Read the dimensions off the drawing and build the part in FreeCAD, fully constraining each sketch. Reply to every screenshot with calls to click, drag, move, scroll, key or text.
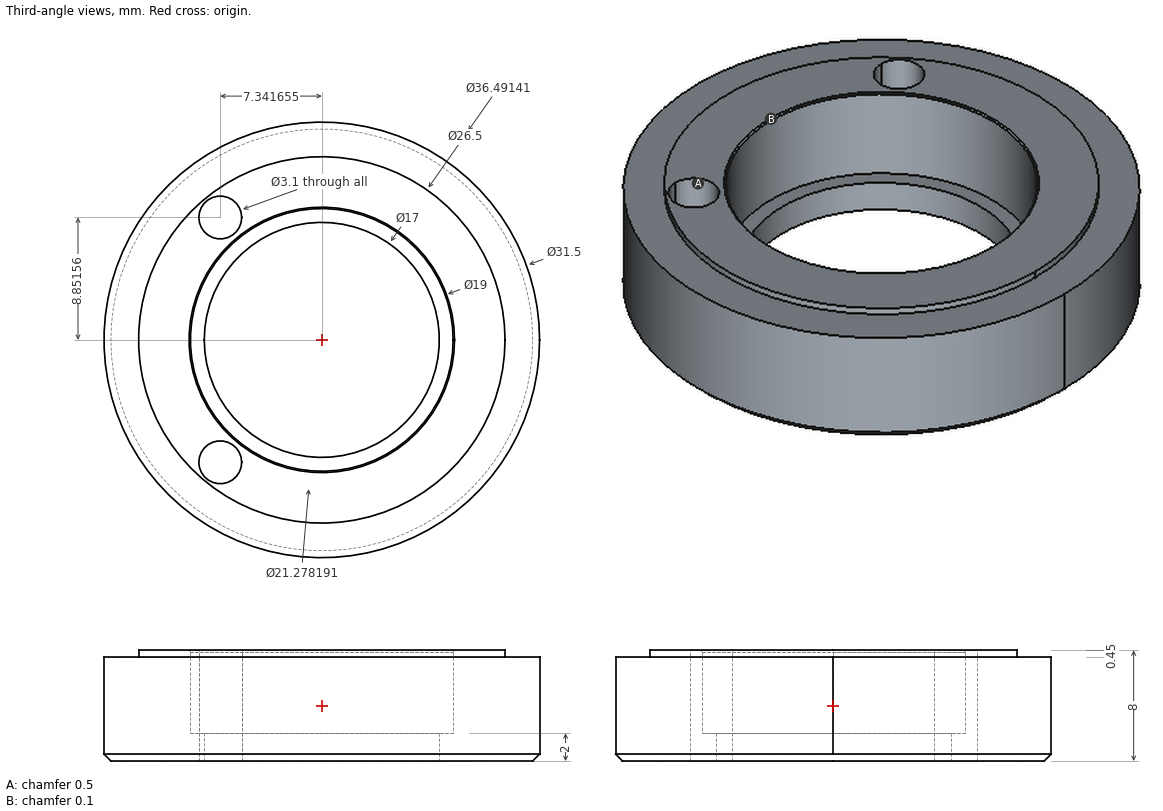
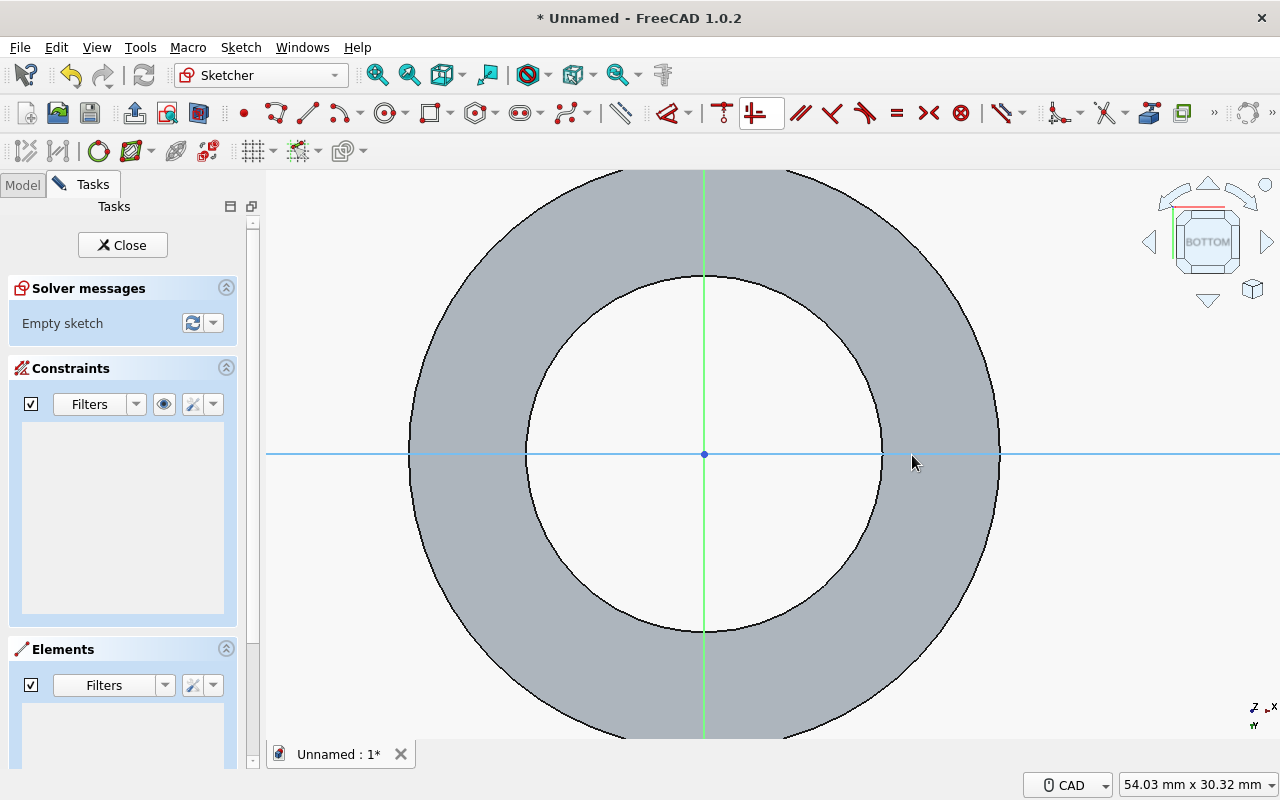
click(386, 114)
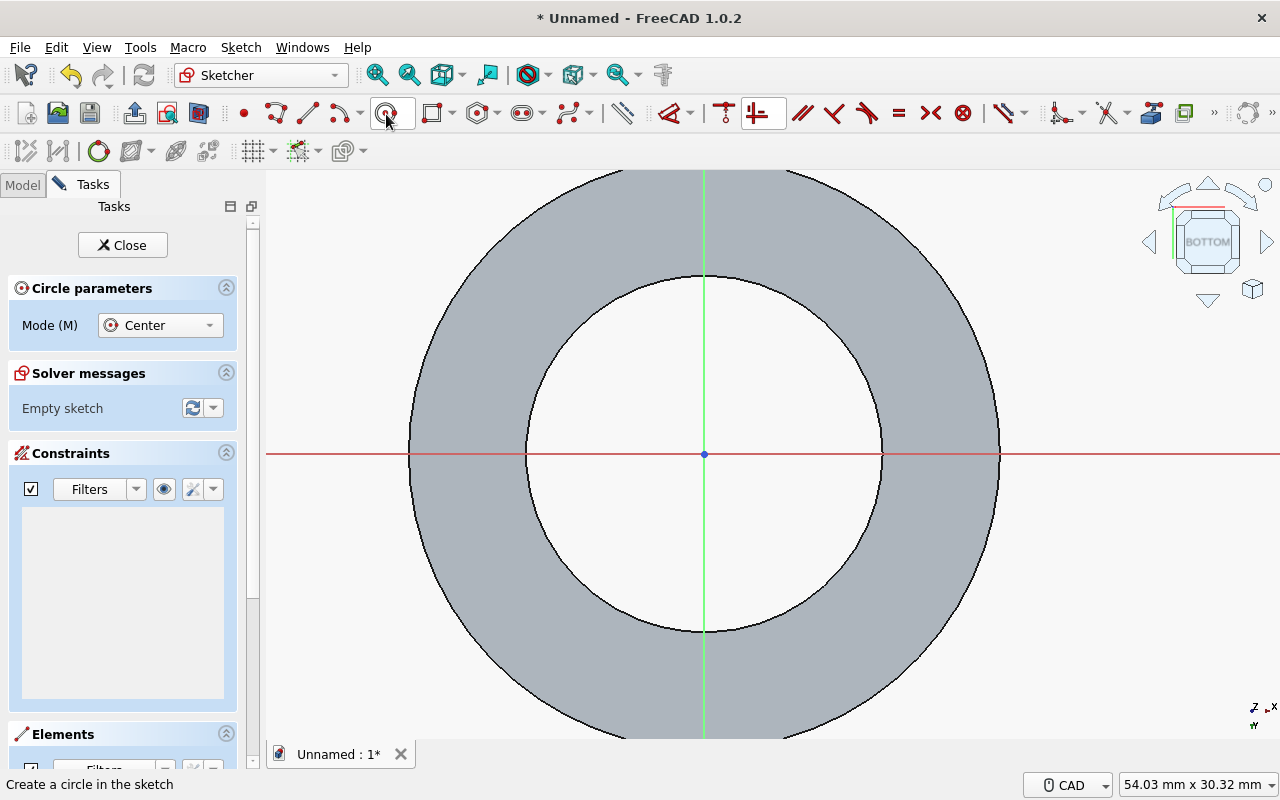
click(704, 454)
move(846, 313)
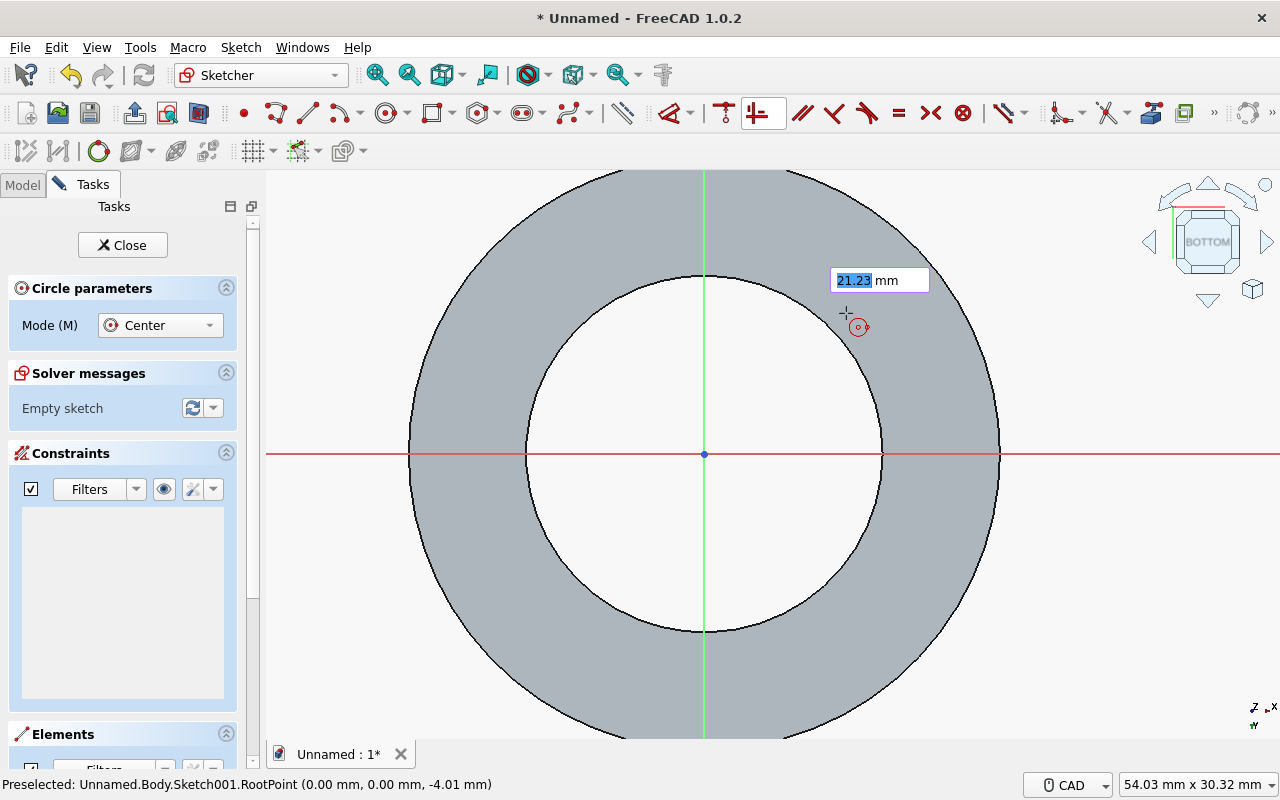
text(21.278191)
key(Return)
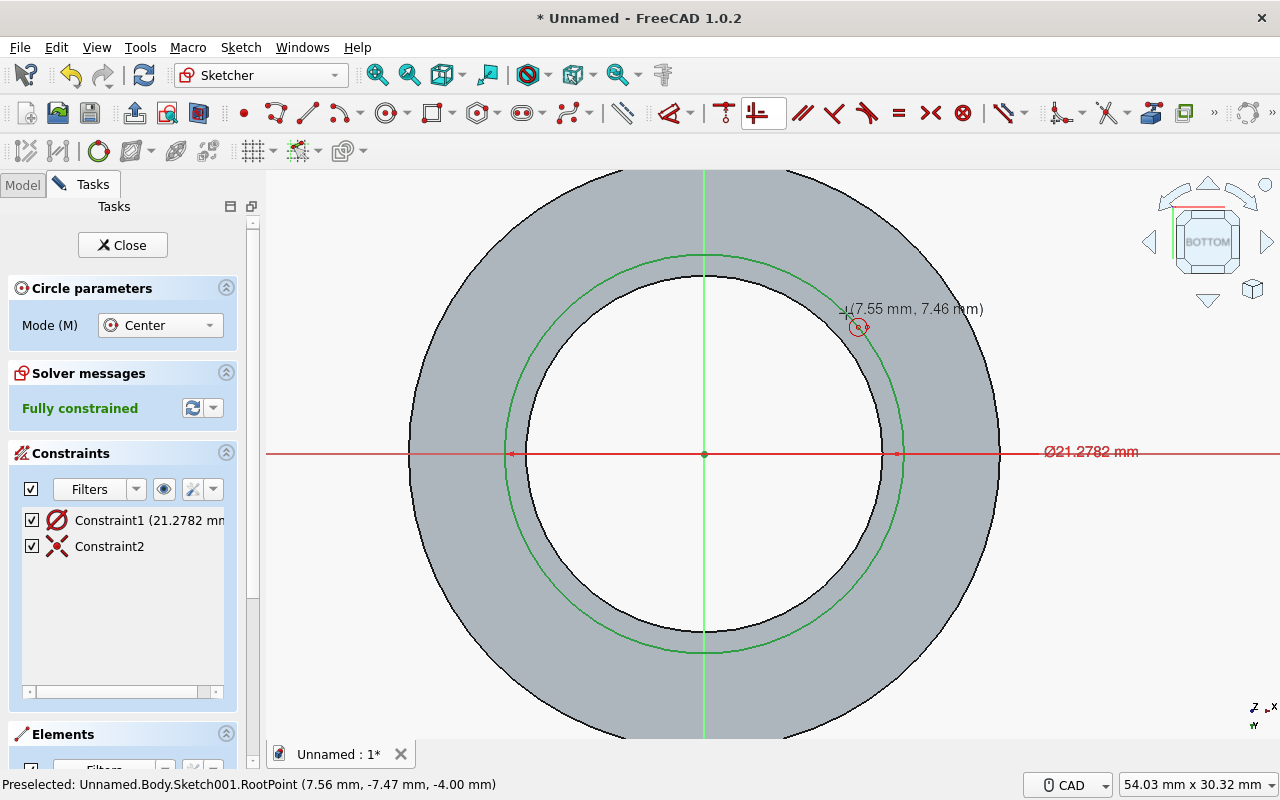
click(704, 454)
move(817, 341)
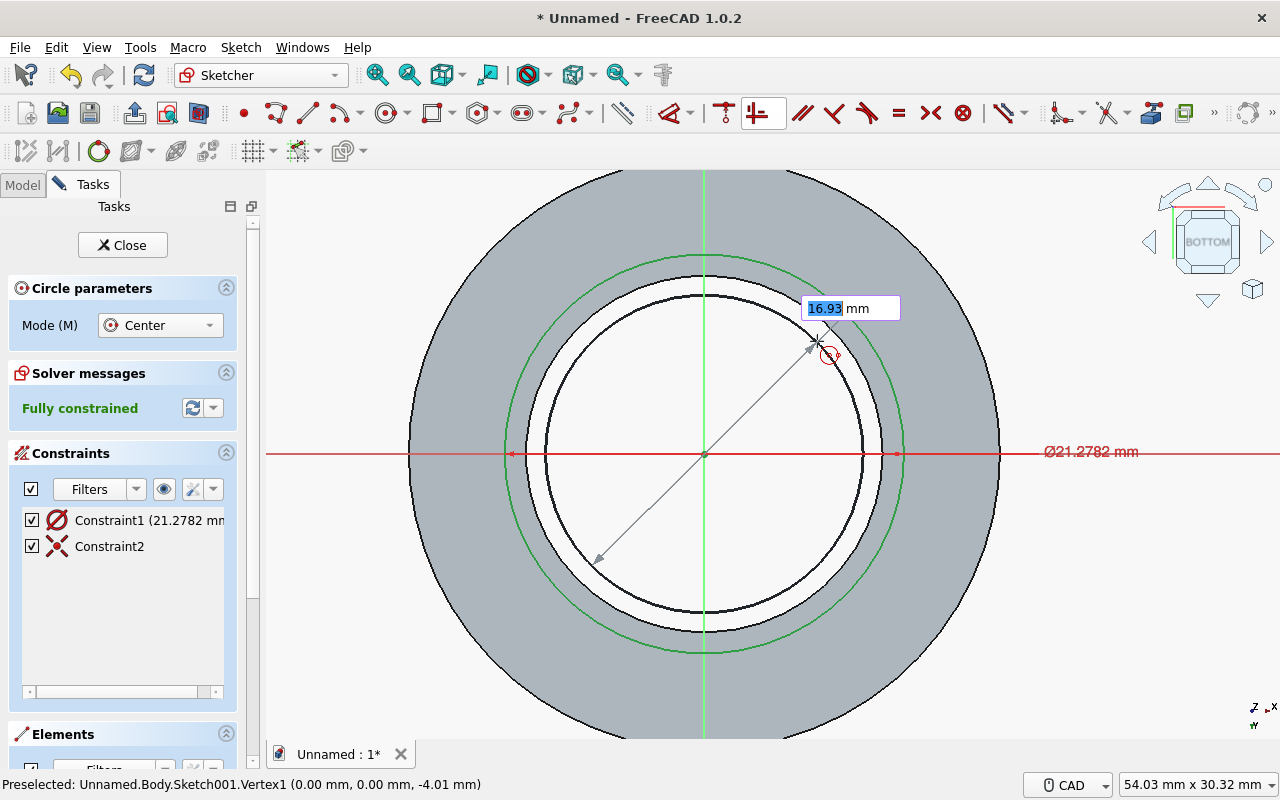
text(17)
key(Return)
key(Escape)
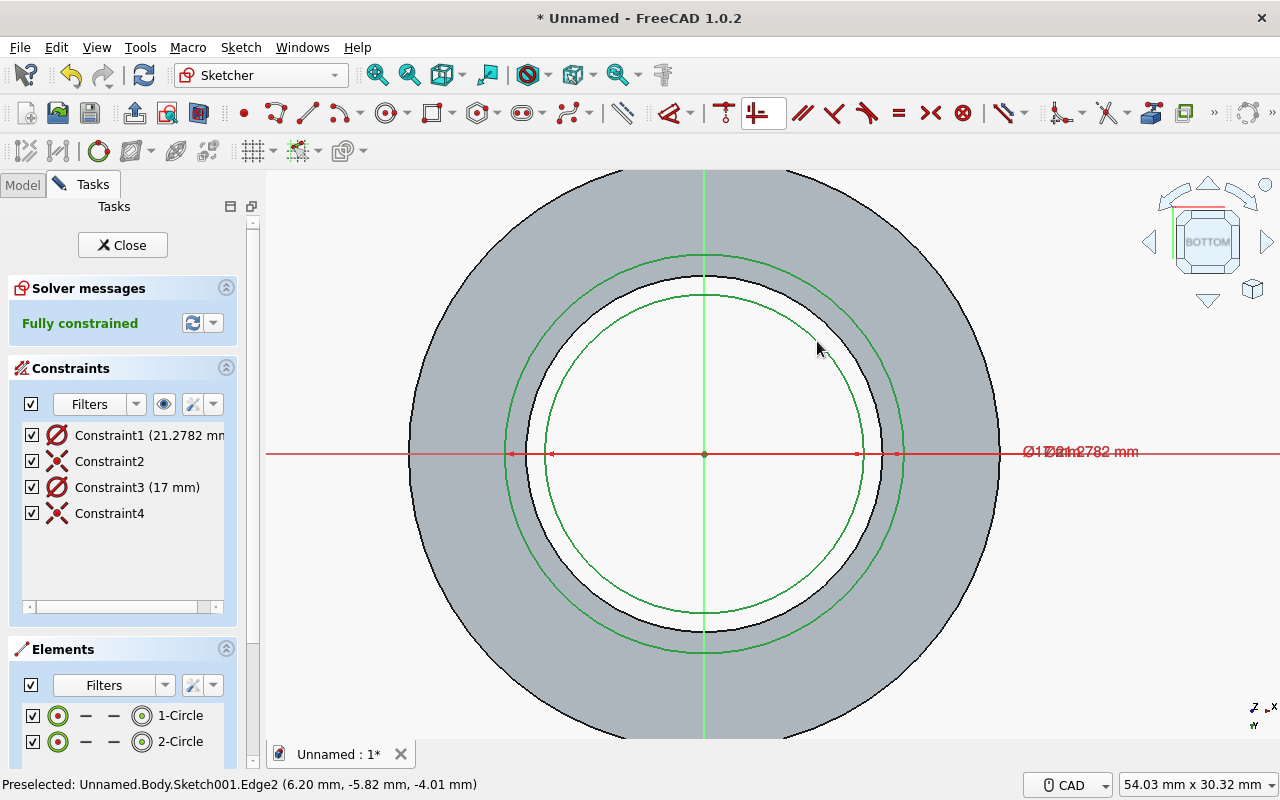
click(123, 245)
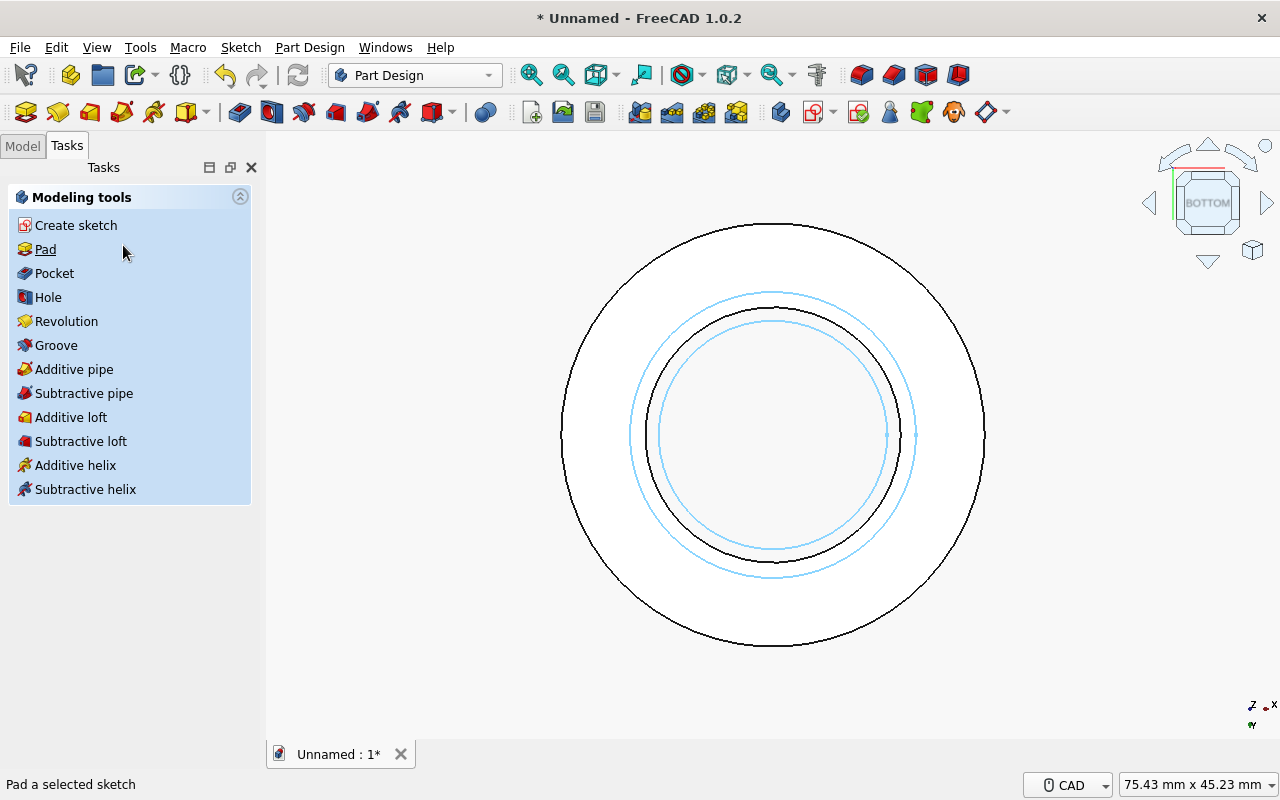
click(26, 112)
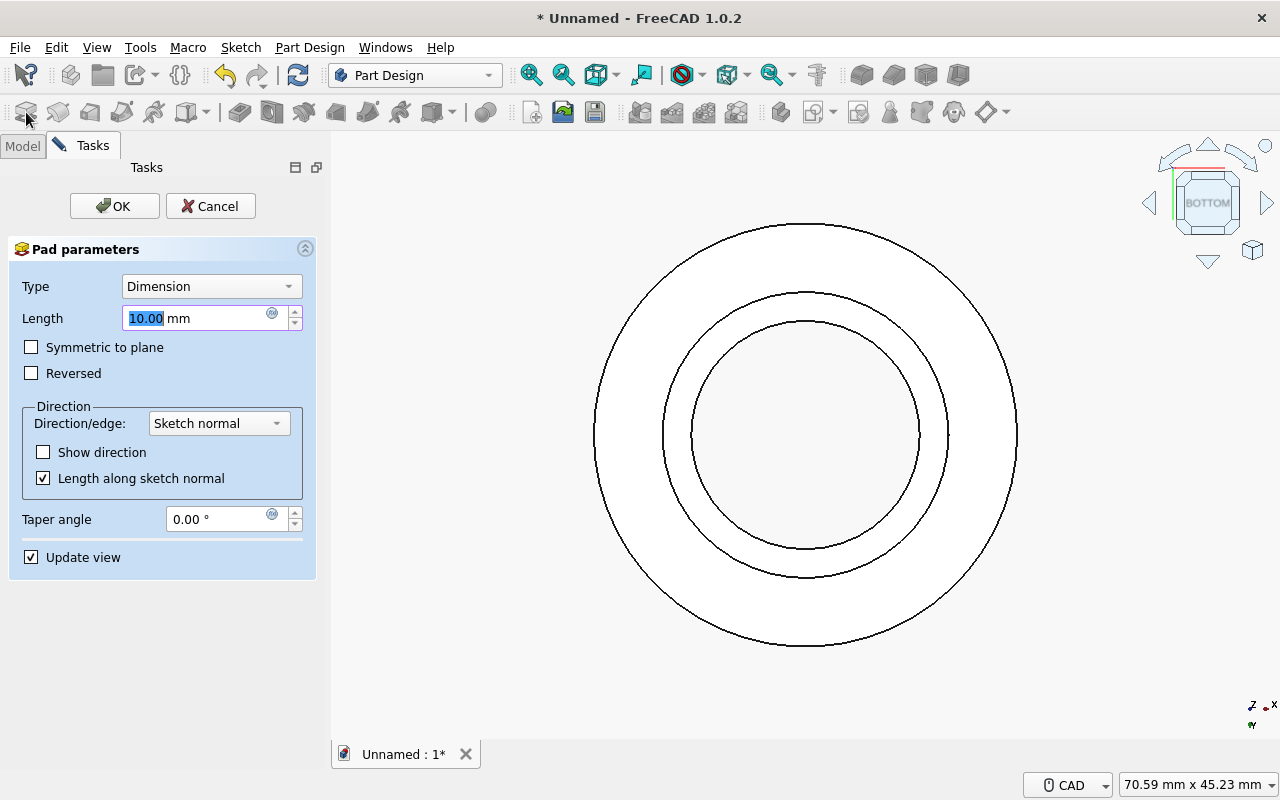
text(2)
key(Tab)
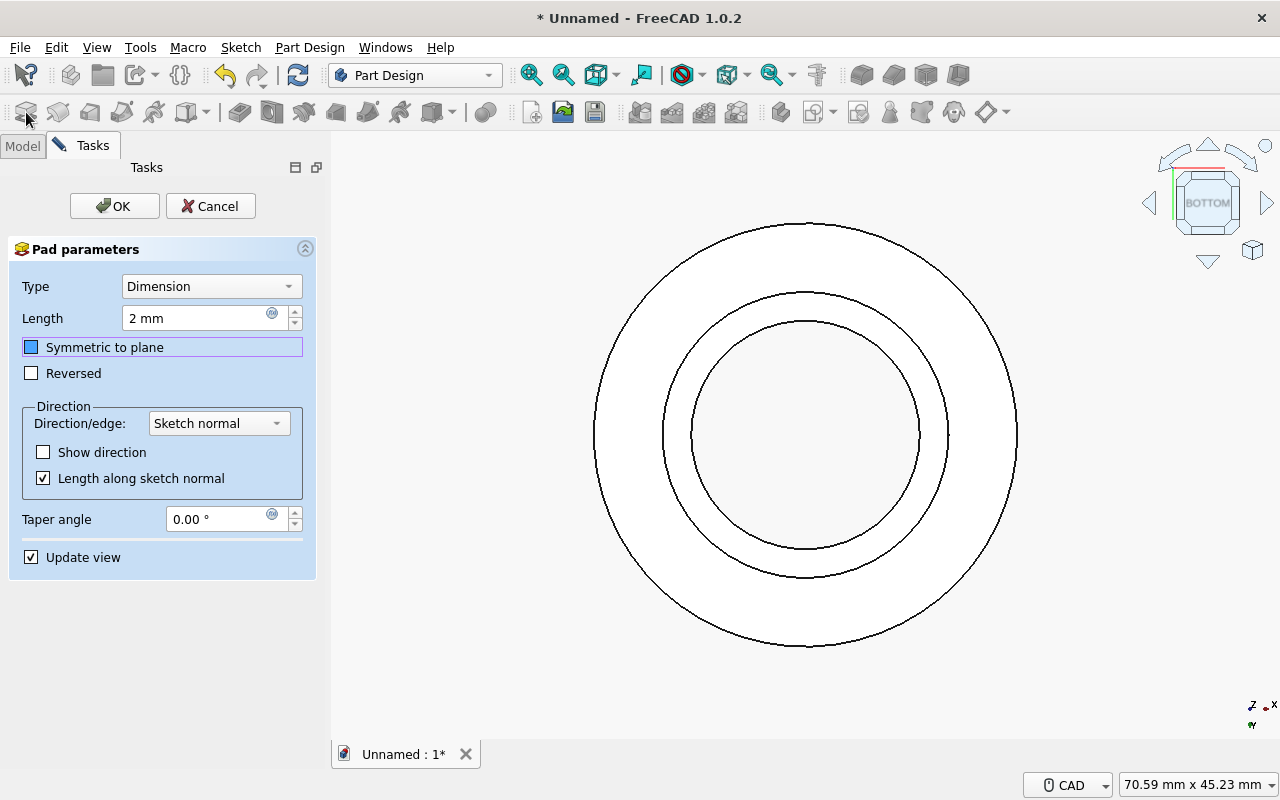
click(30, 373)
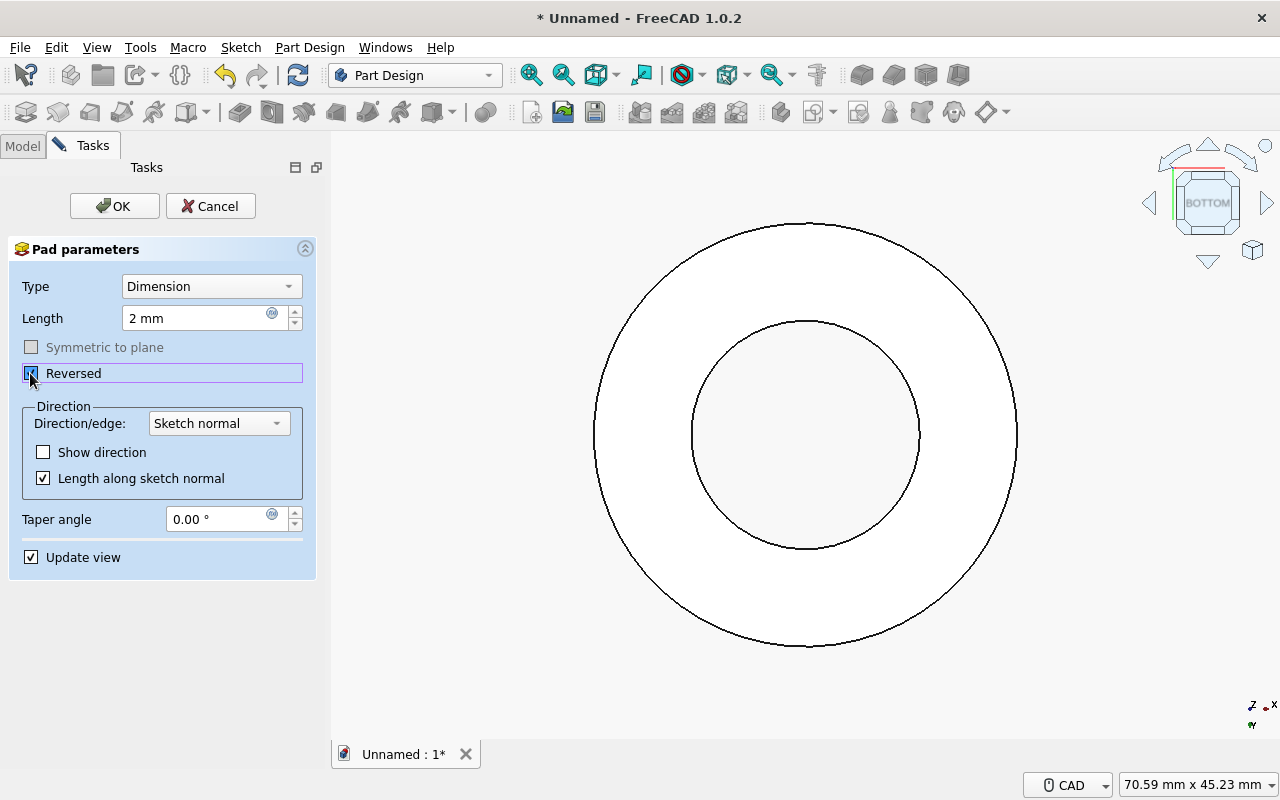
click(115, 206)